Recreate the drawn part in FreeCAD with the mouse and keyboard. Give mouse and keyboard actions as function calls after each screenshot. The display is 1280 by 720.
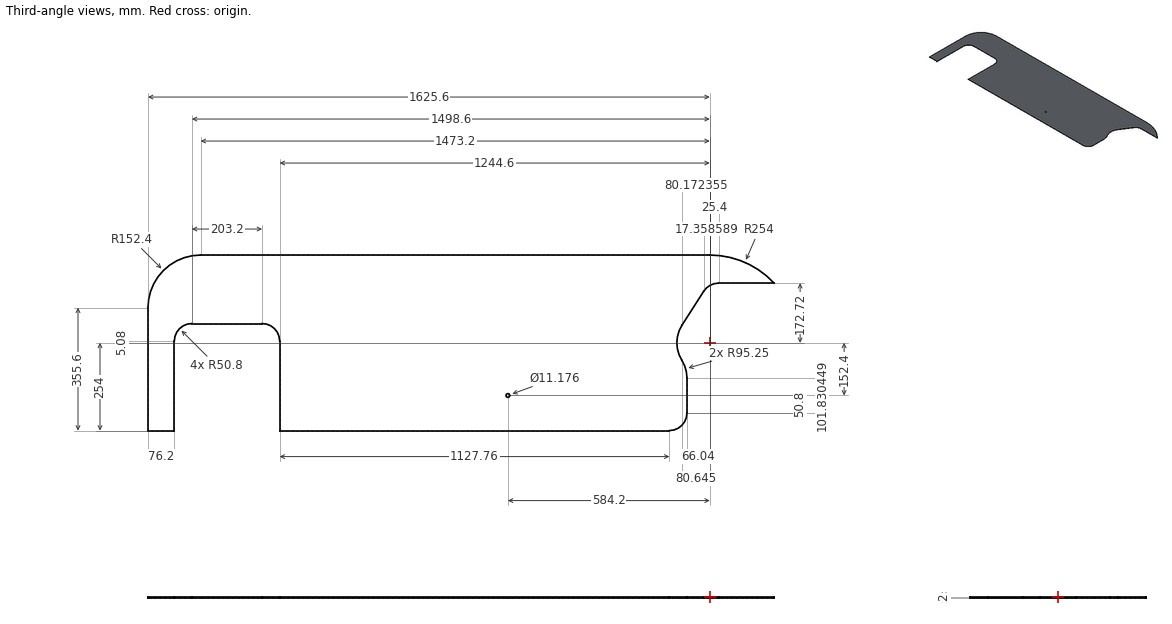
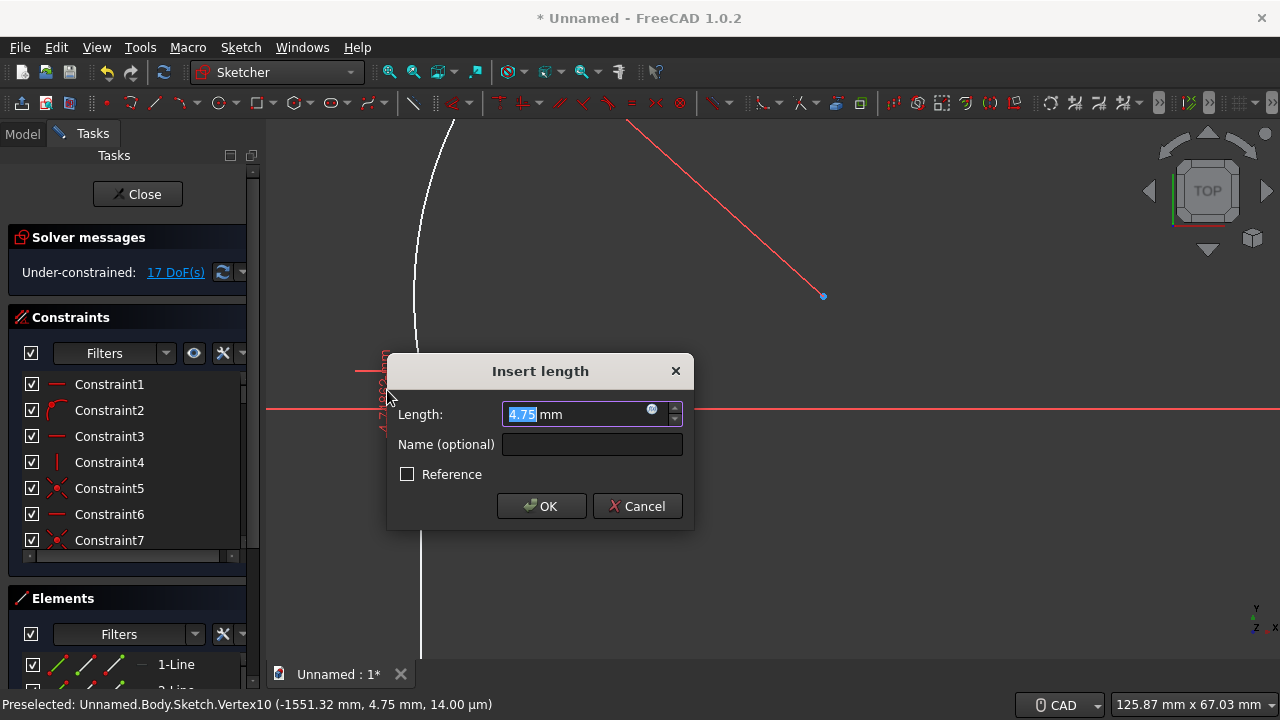
text(5.08)
key(Return)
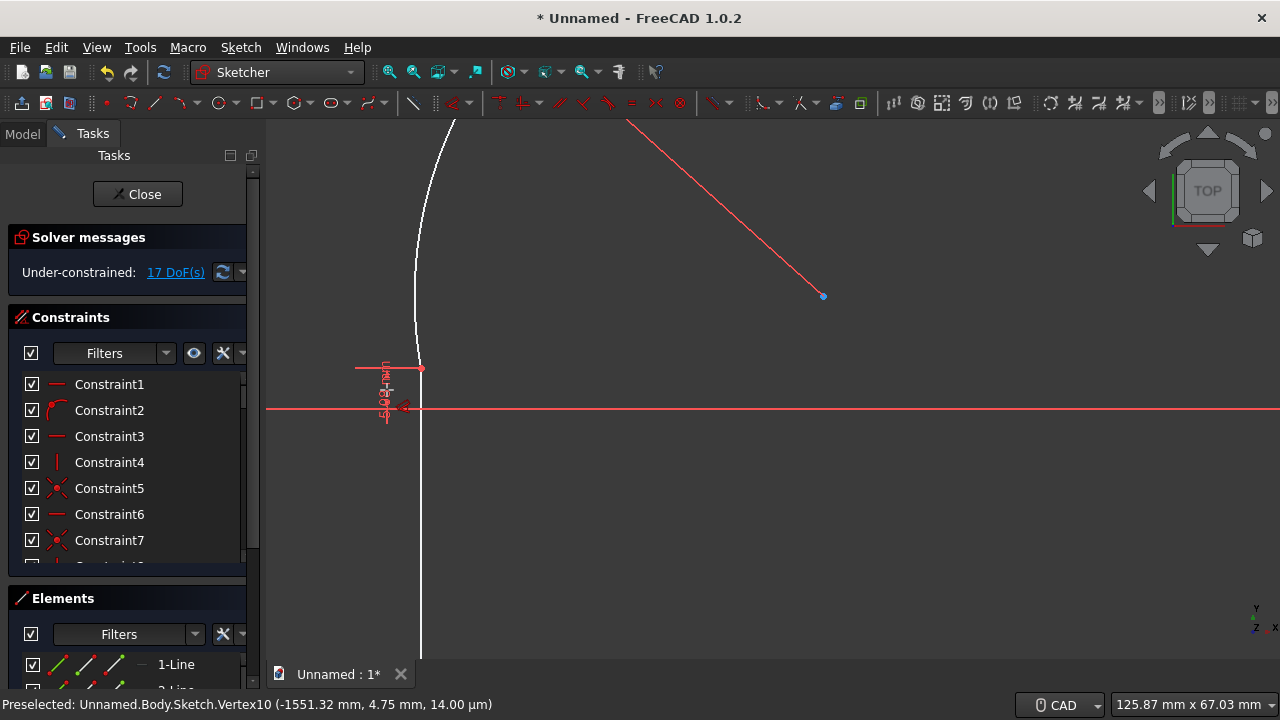
scroll(368, 388, down, 15)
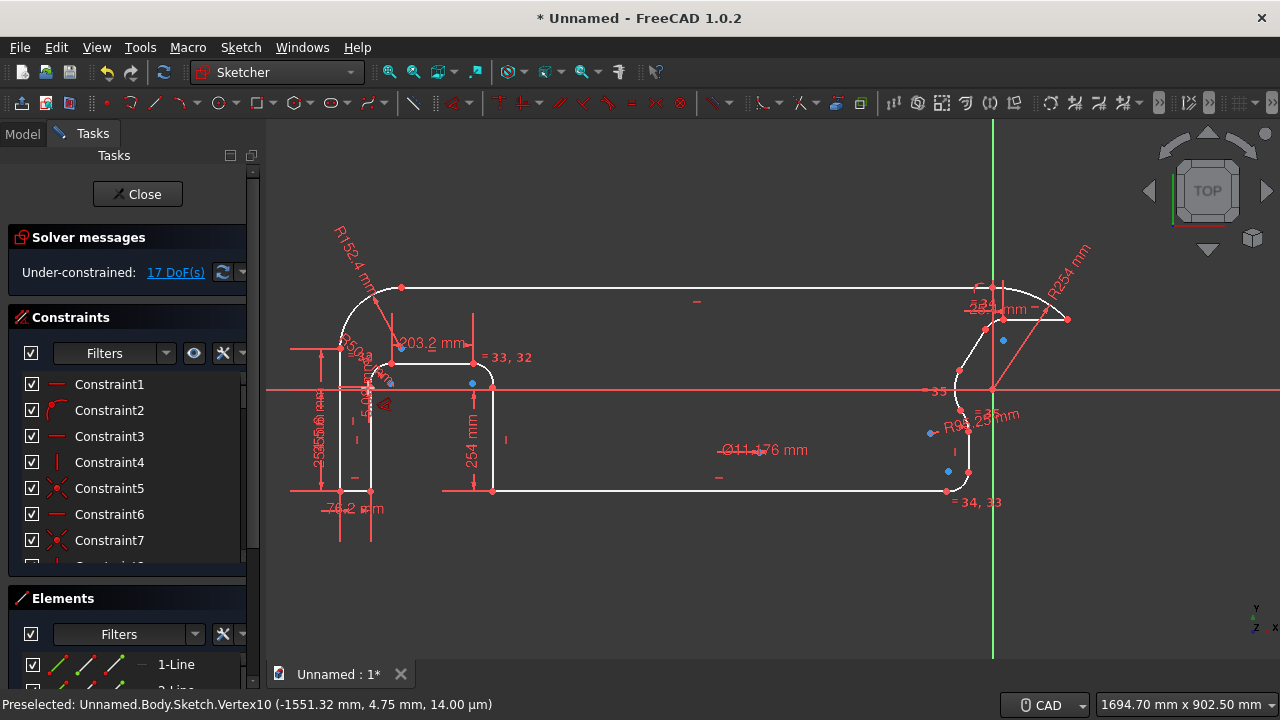
scroll(493, 388, up, 15)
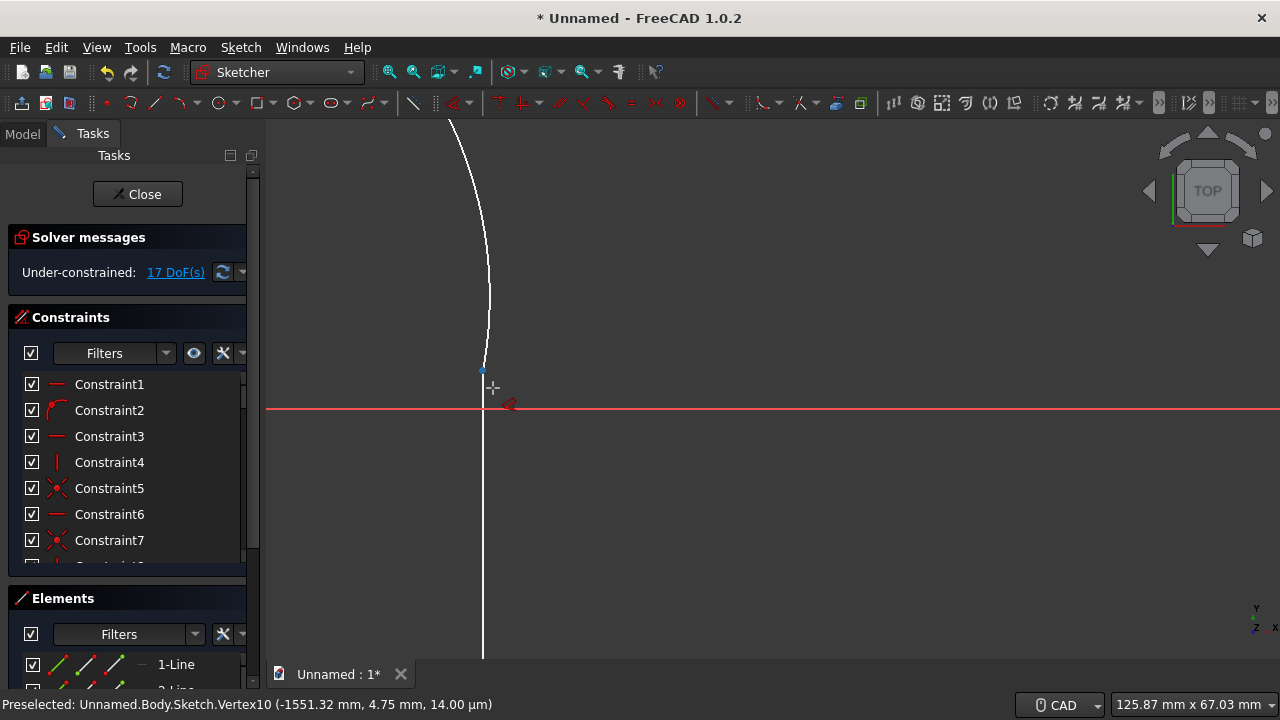
click(483, 371)
click(449, 390)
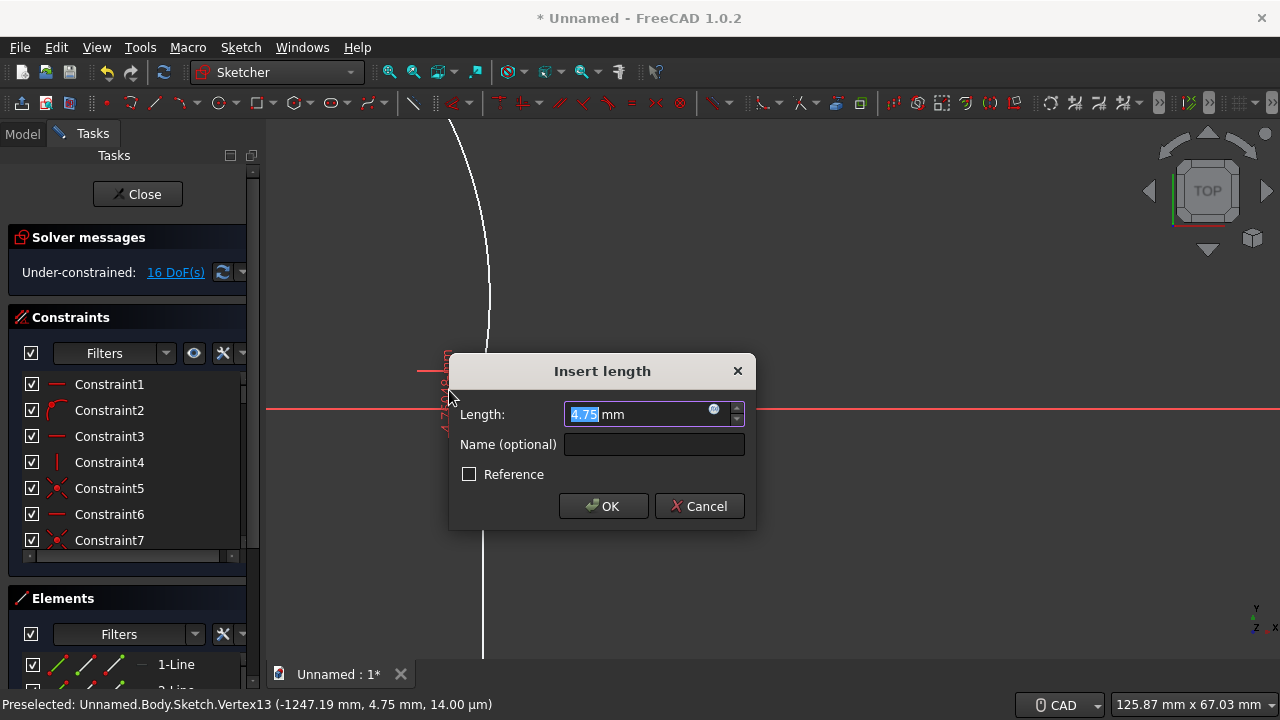
text(5.08)
key(Return)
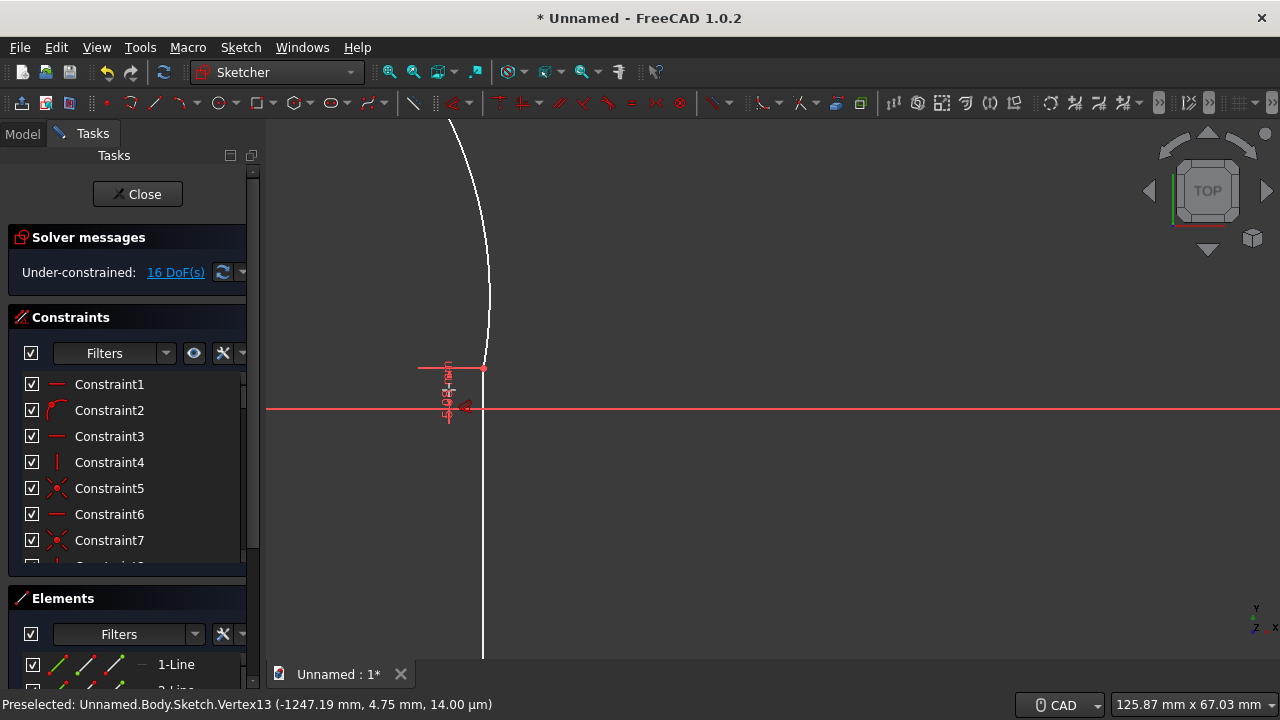
scroll(493, 388, down, 15)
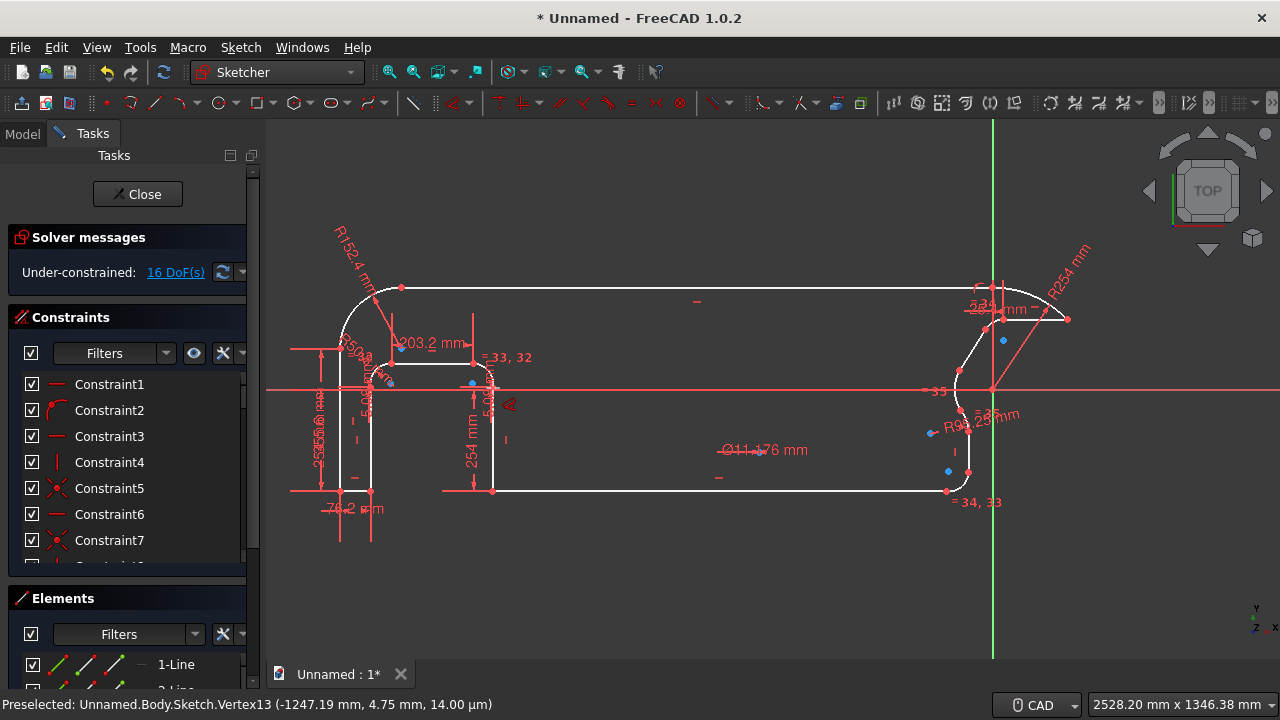
scroll(391, 384, up, 15)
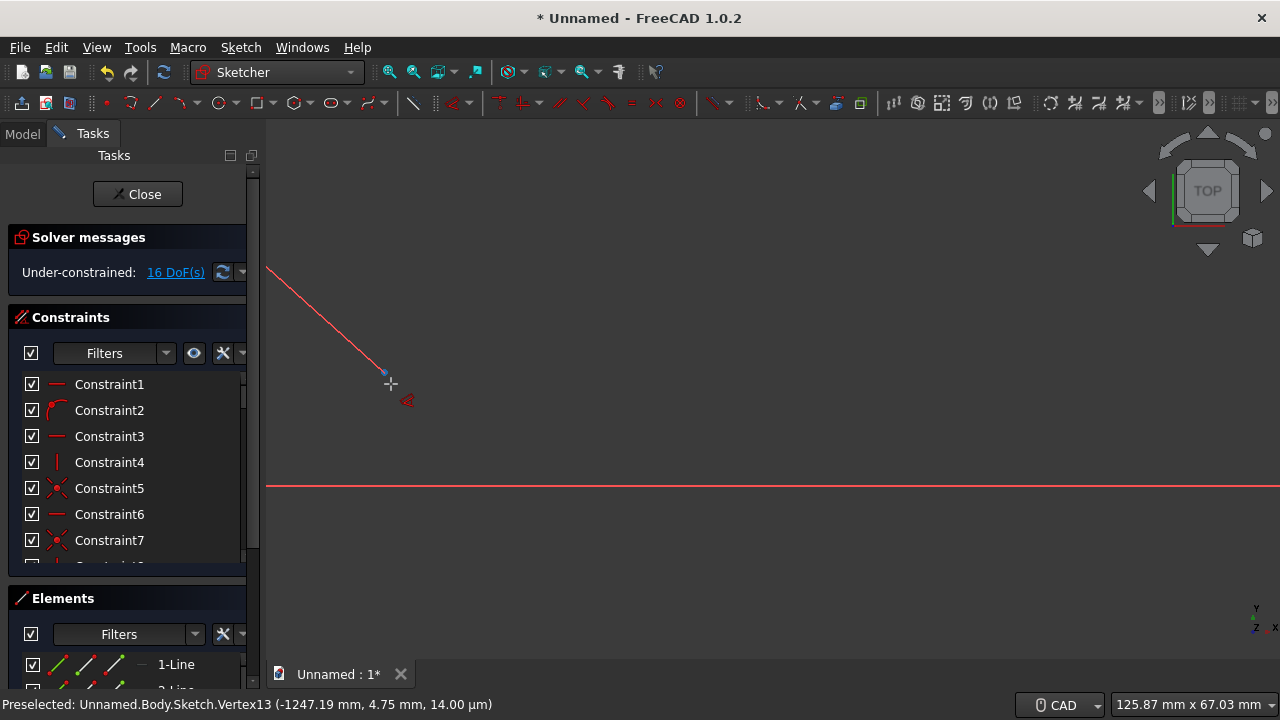
click(384, 373)
click(350, 429)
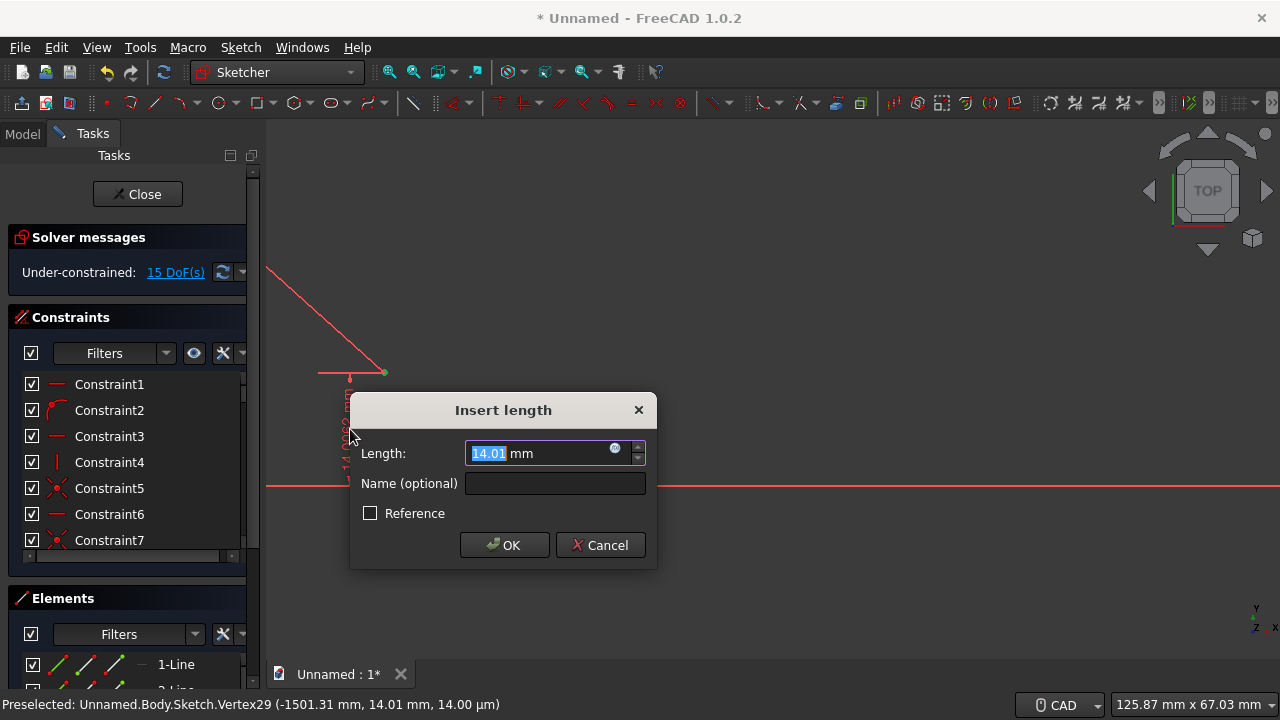
text(5.08)
key(Return)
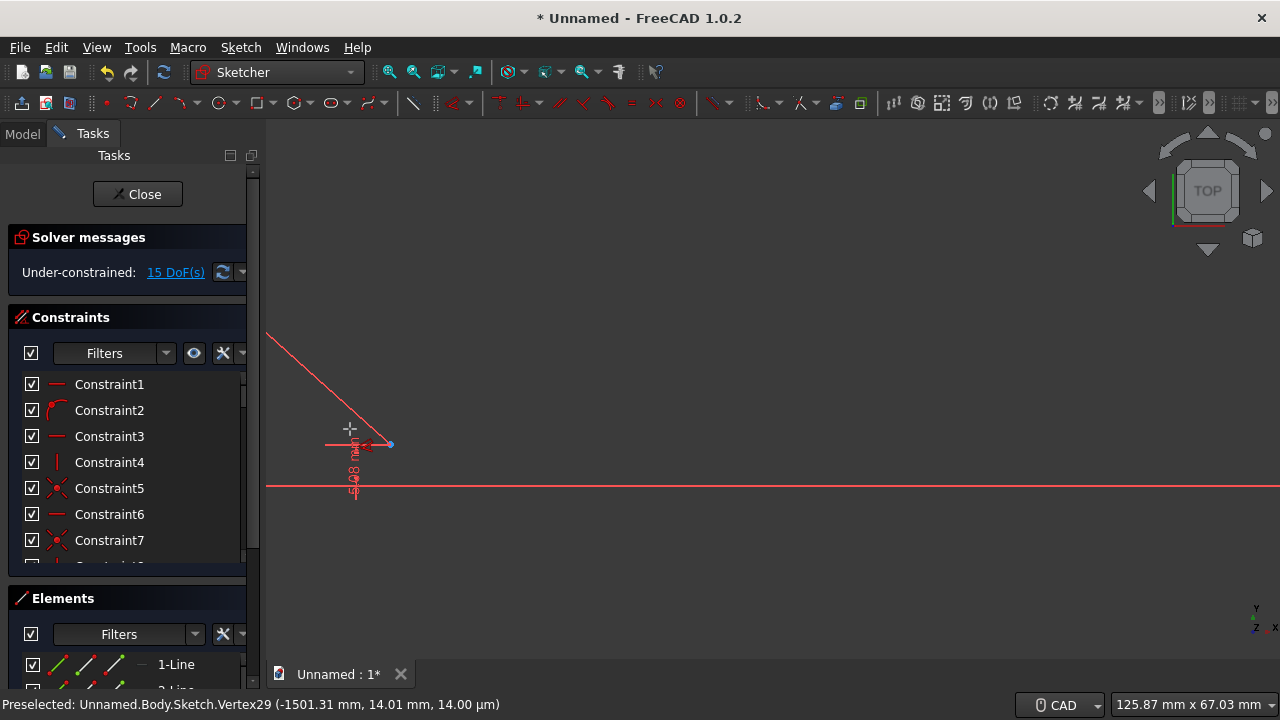
scroll(391, 384, down, 15)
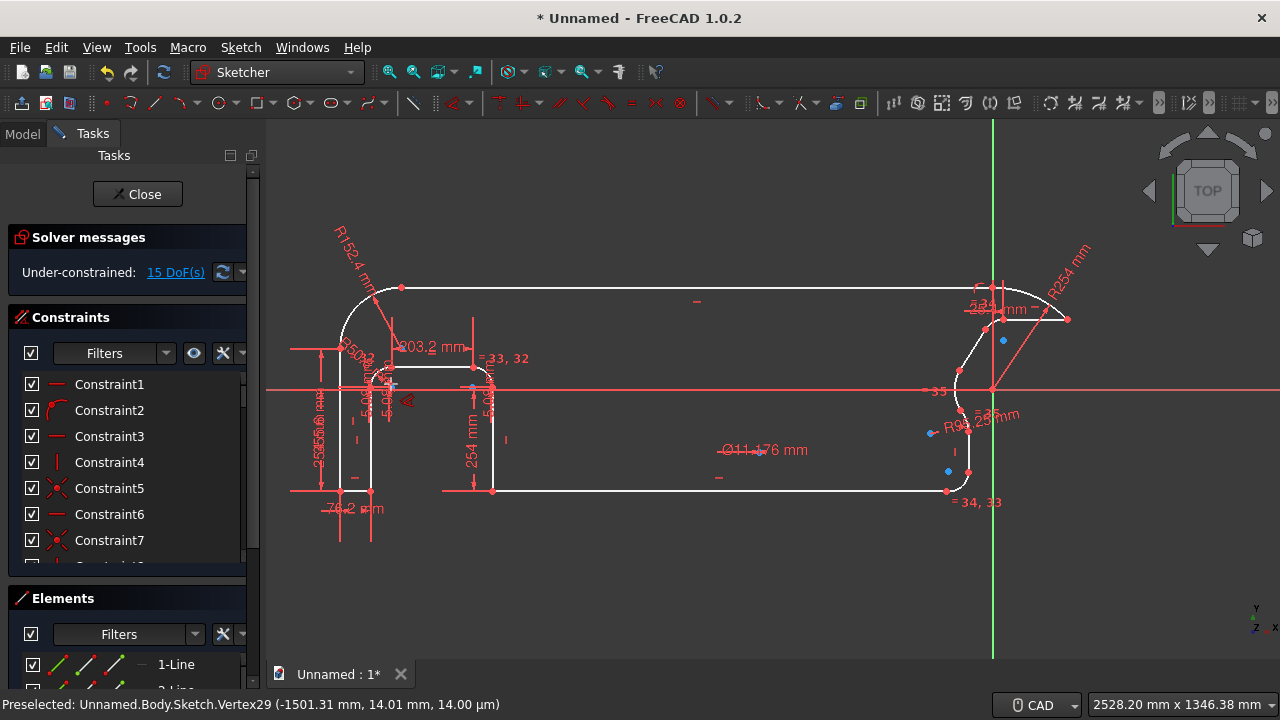
scroll(1003, 340, up, 7)